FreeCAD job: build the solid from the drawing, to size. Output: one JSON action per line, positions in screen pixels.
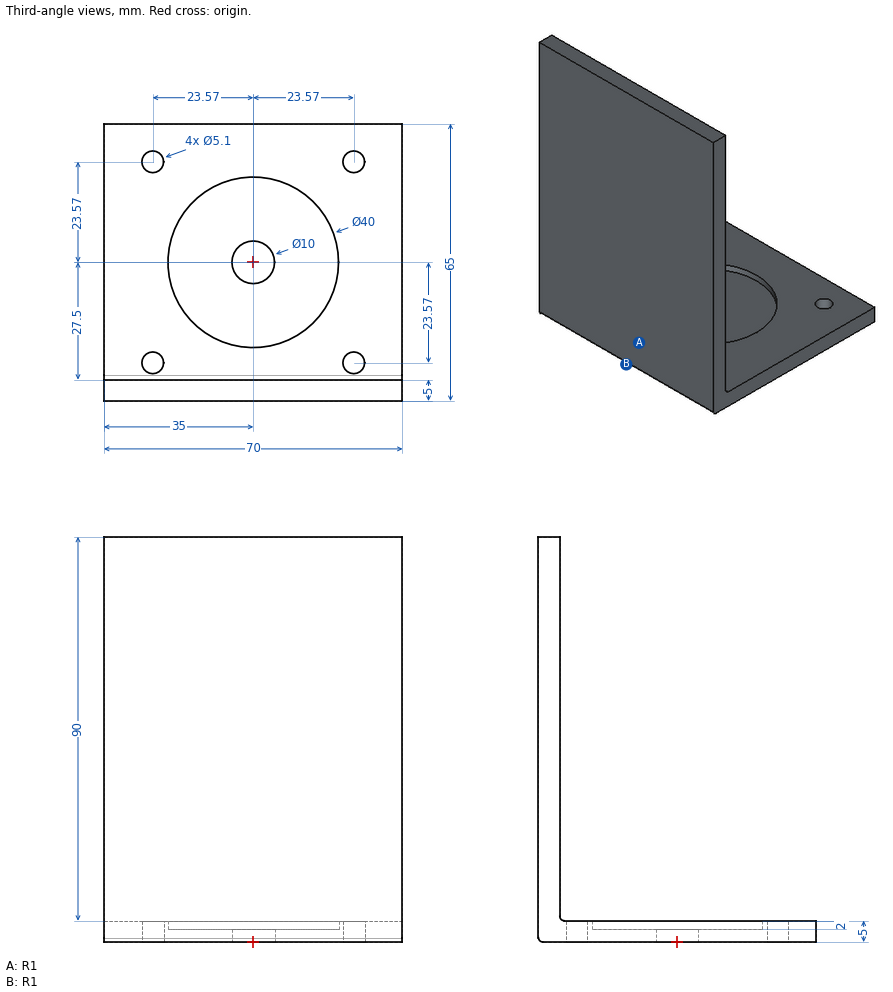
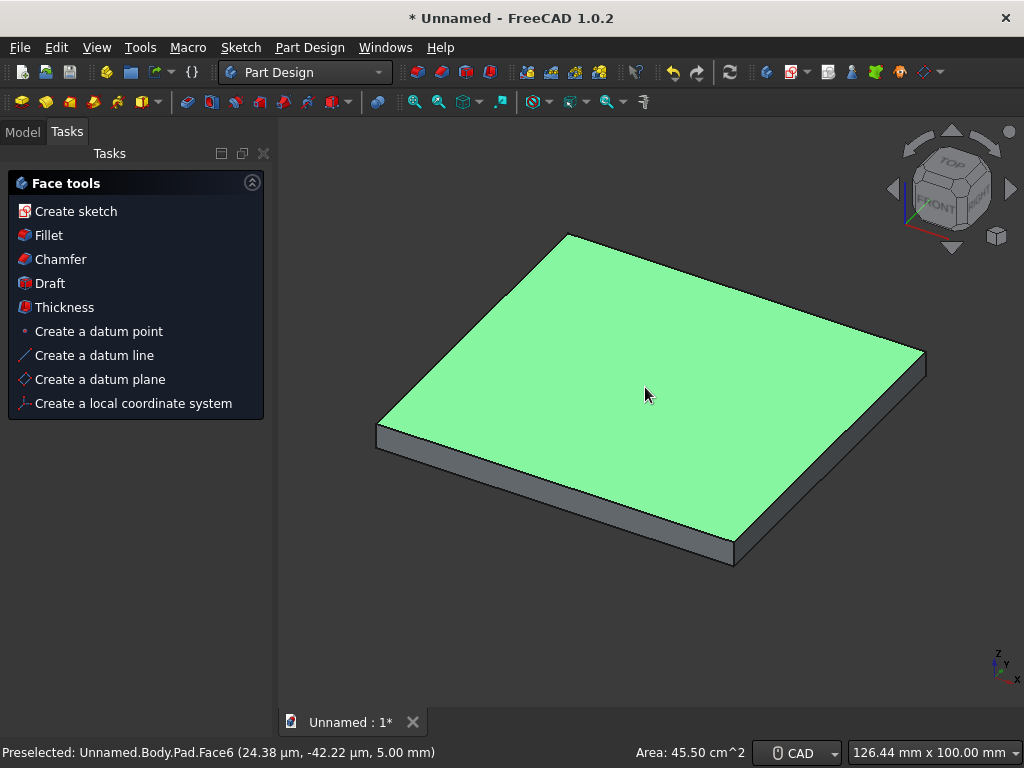
{"action": "left_click", "coordinate": [792, 72]}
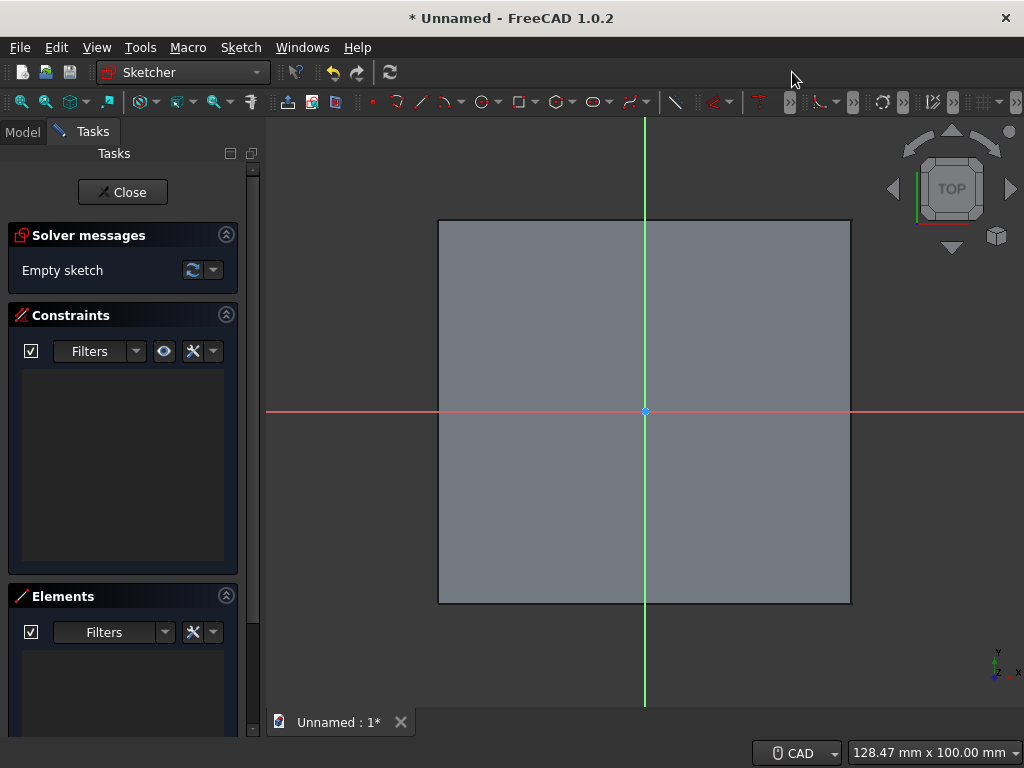
{"action": "left_click", "coordinate": [482, 102]}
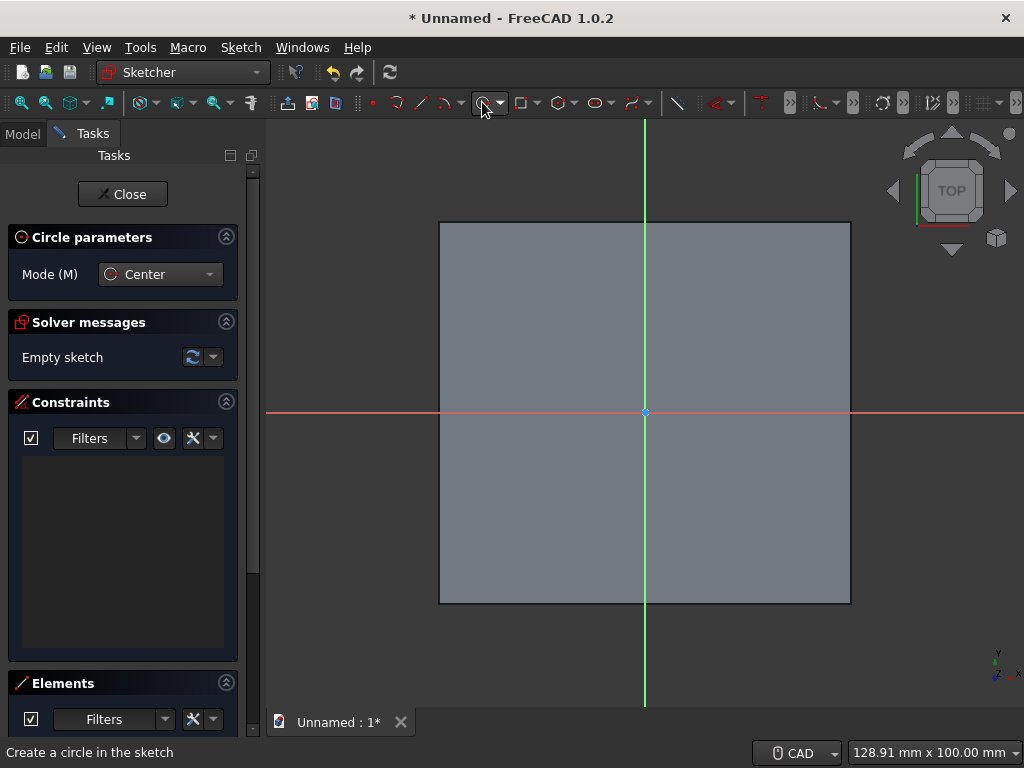
{"action": "scroll", "coordinate": [506, 274], "scroll_direction": "up", "scroll_amount": 3}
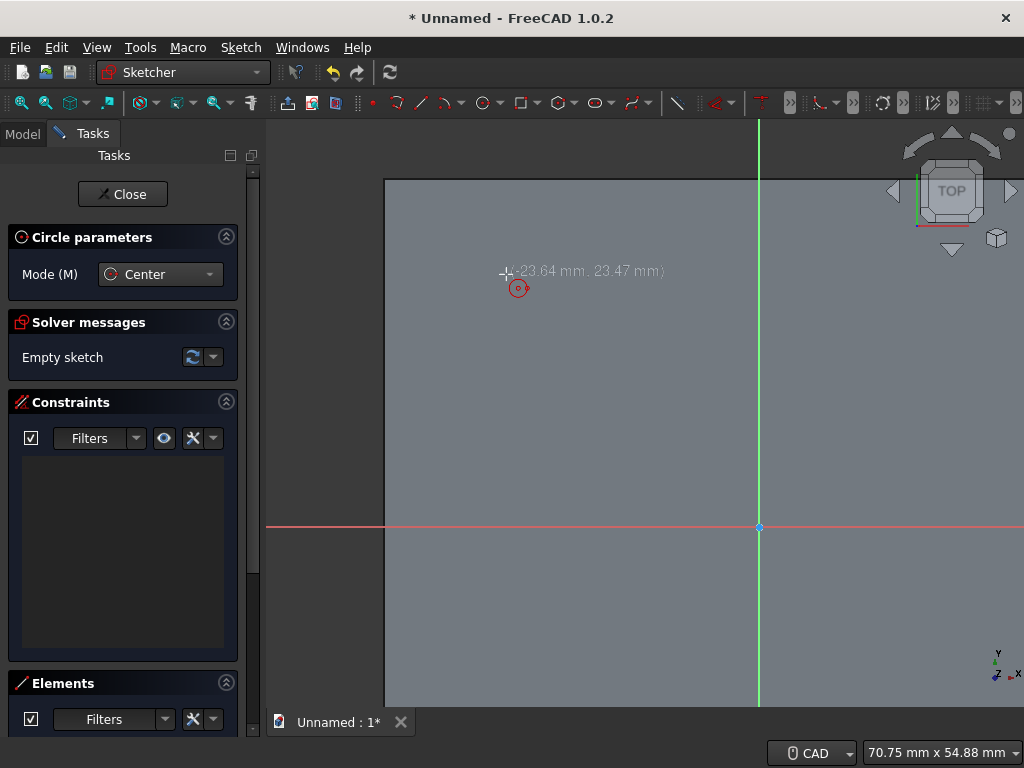
{"action": "left_click", "coordinate": [506, 275]}
{"action": "mouse_move", "coordinate": [526, 255]}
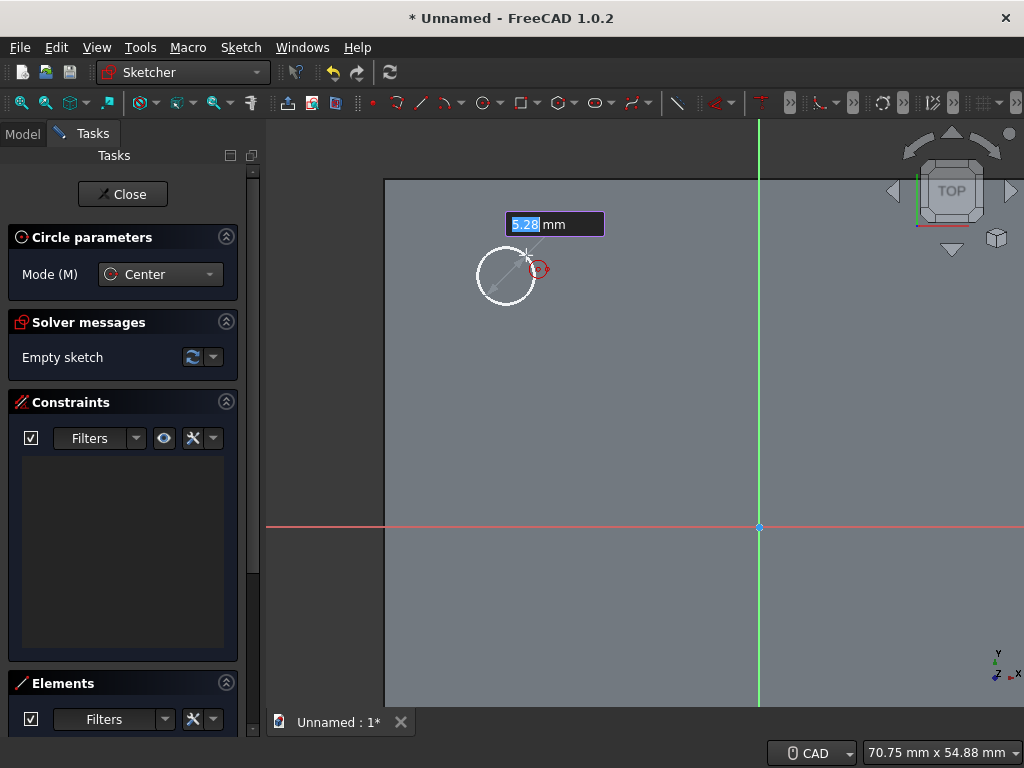
{"action": "type", "text": "5.1"}
{"action": "key", "text": "Return"}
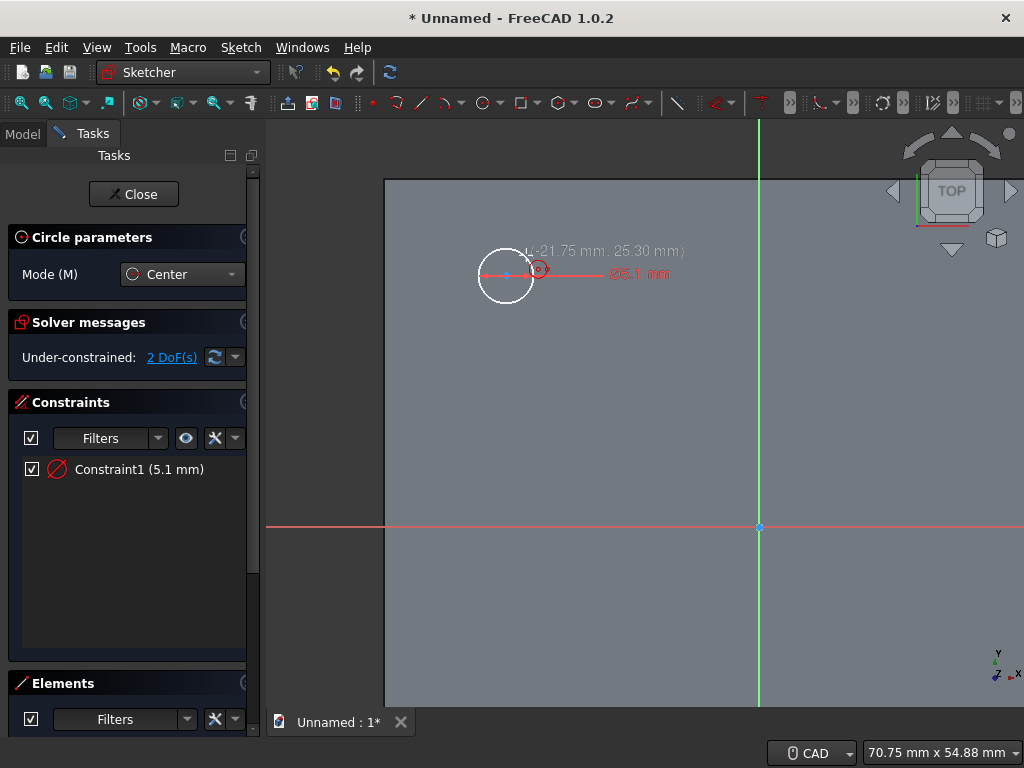
{"action": "scroll", "coordinate": [294, 181], "scroll_direction": "down", "scroll_amount": 2}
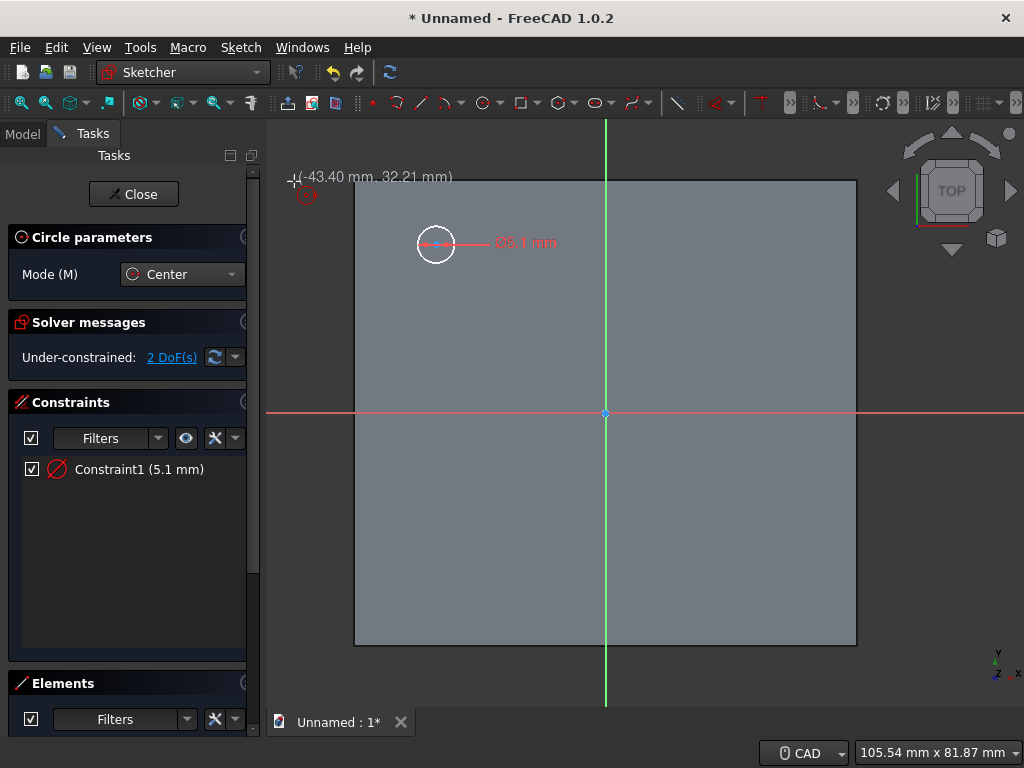
{"action": "scroll", "coordinate": [775, 244], "scroll_direction": "up", "scroll_amount": 2}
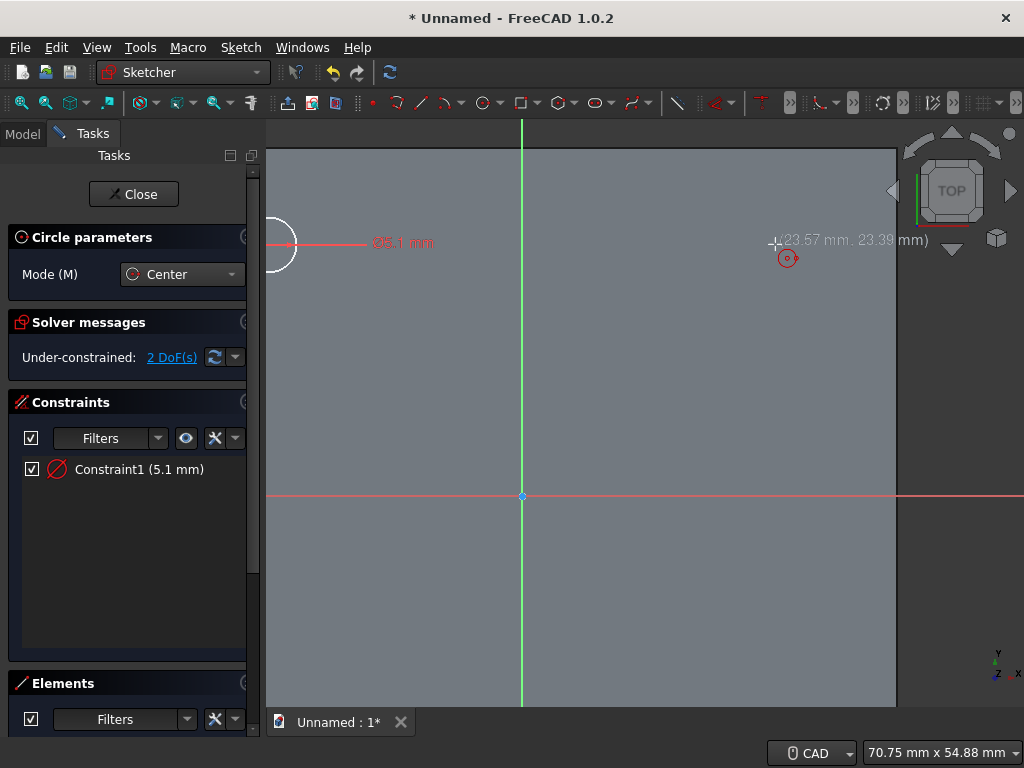
{"action": "left_click", "coordinate": [775, 243]}
{"action": "mouse_move", "coordinate": [794, 224]}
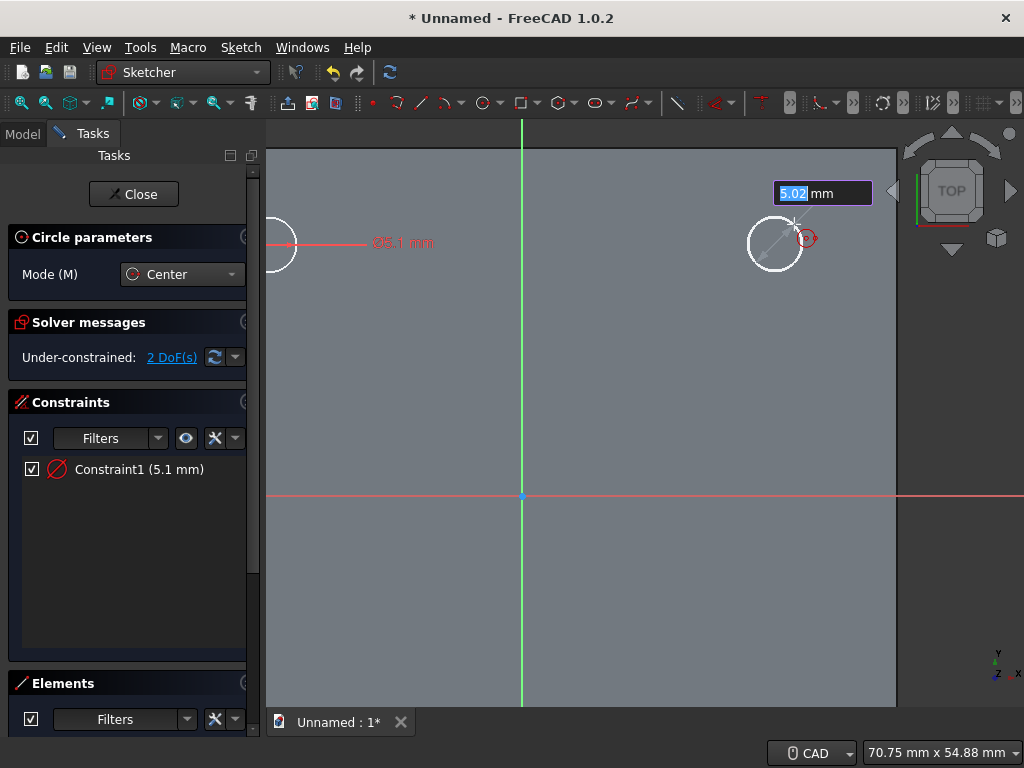
{"action": "type", "text": "5.1"}
{"action": "key", "text": "Return"}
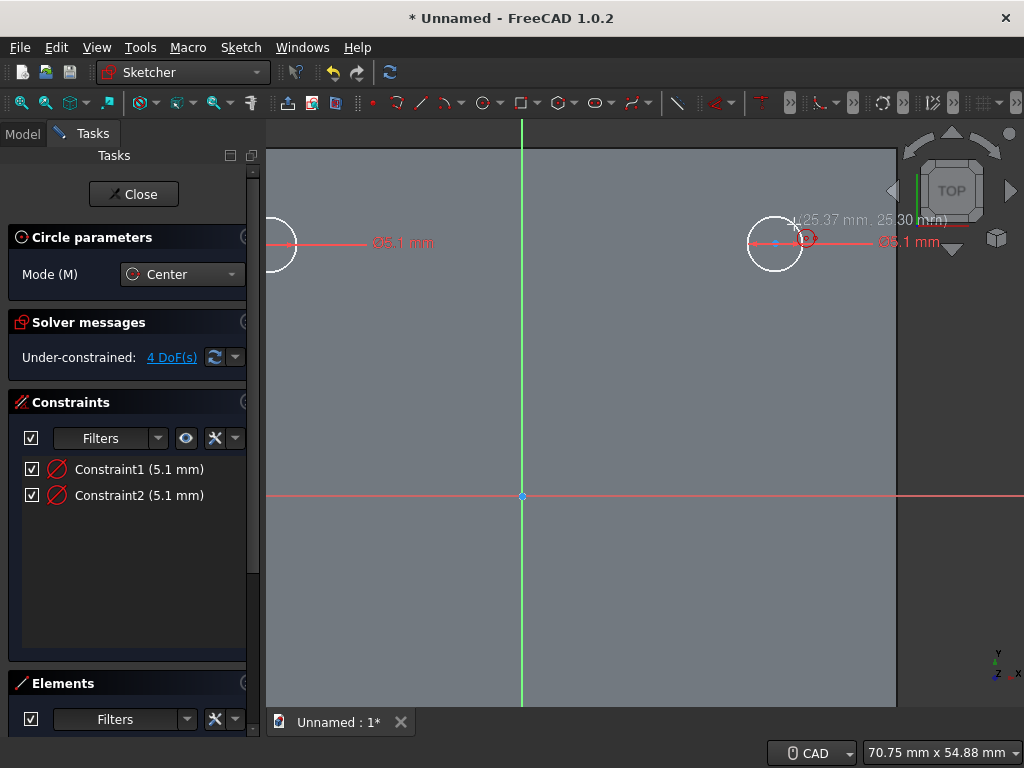
{"action": "scroll", "coordinate": [687, 244], "scroll_direction": "down", "scroll_amount": 2}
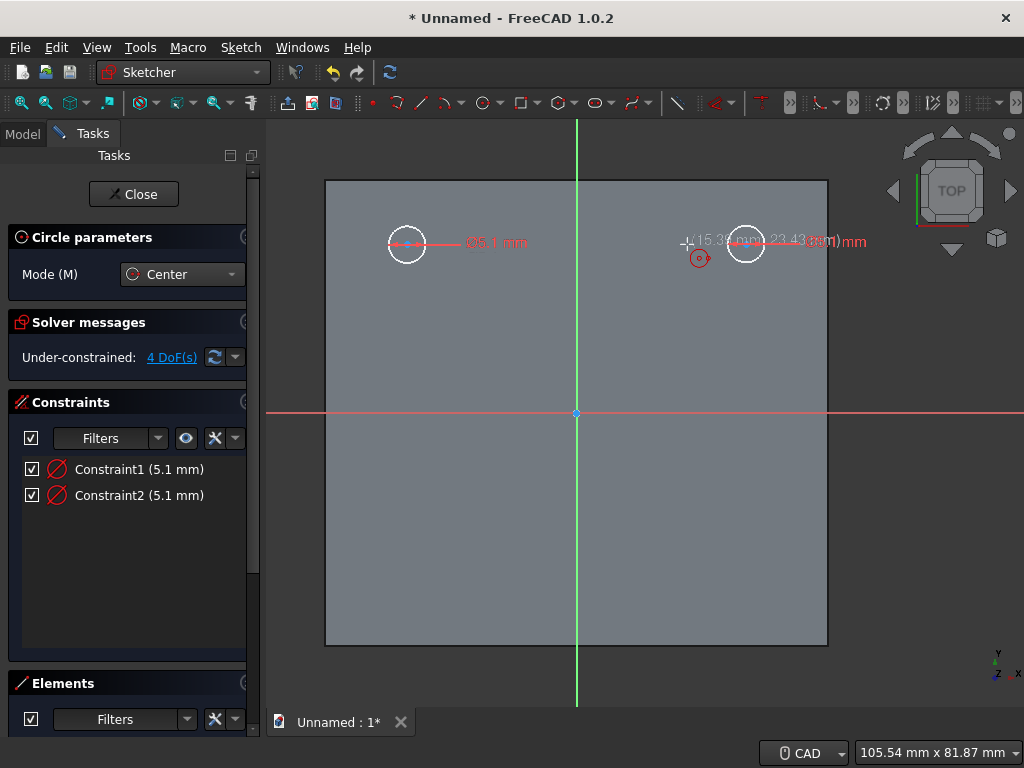
{"action": "scroll", "coordinate": [746, 582], "scroll_direction": "up", "scroll_amount": 2}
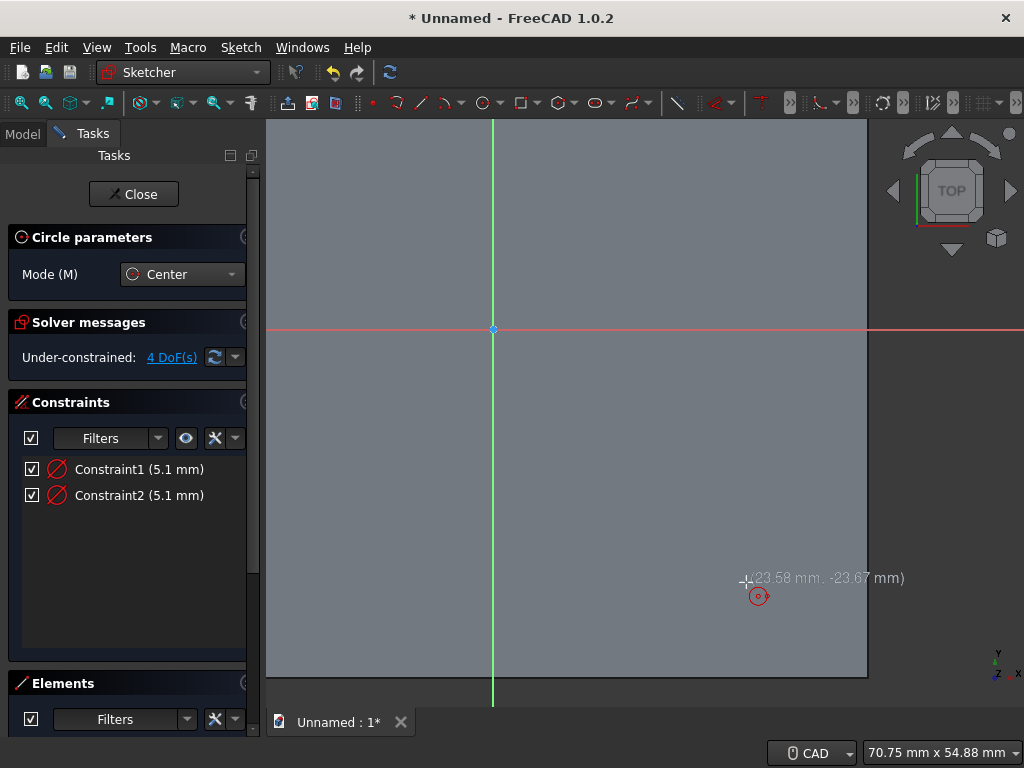
{"action": "left_click", "coordinate": [746, 582]}
{"action": "mouse_move", "coordinate": [765, 563]}